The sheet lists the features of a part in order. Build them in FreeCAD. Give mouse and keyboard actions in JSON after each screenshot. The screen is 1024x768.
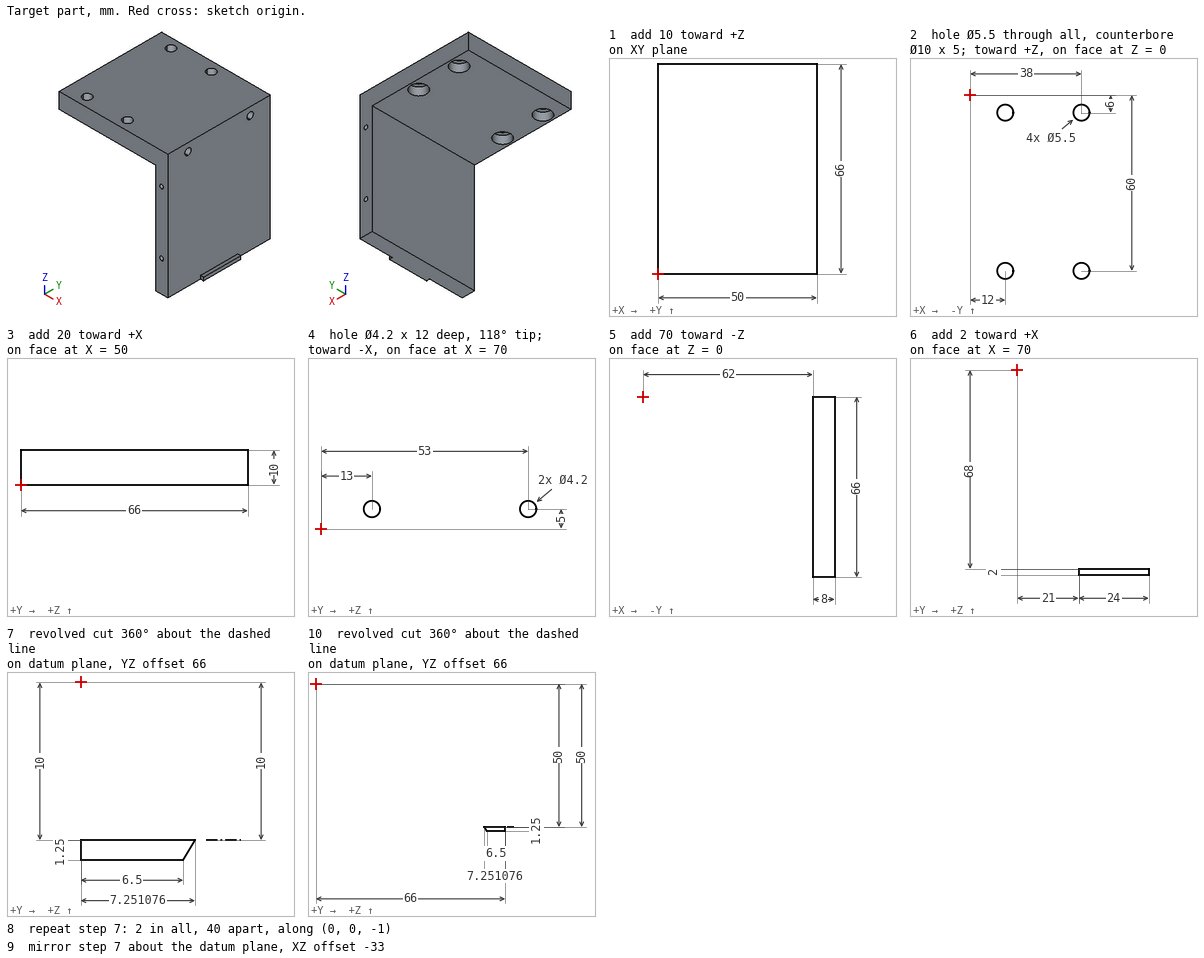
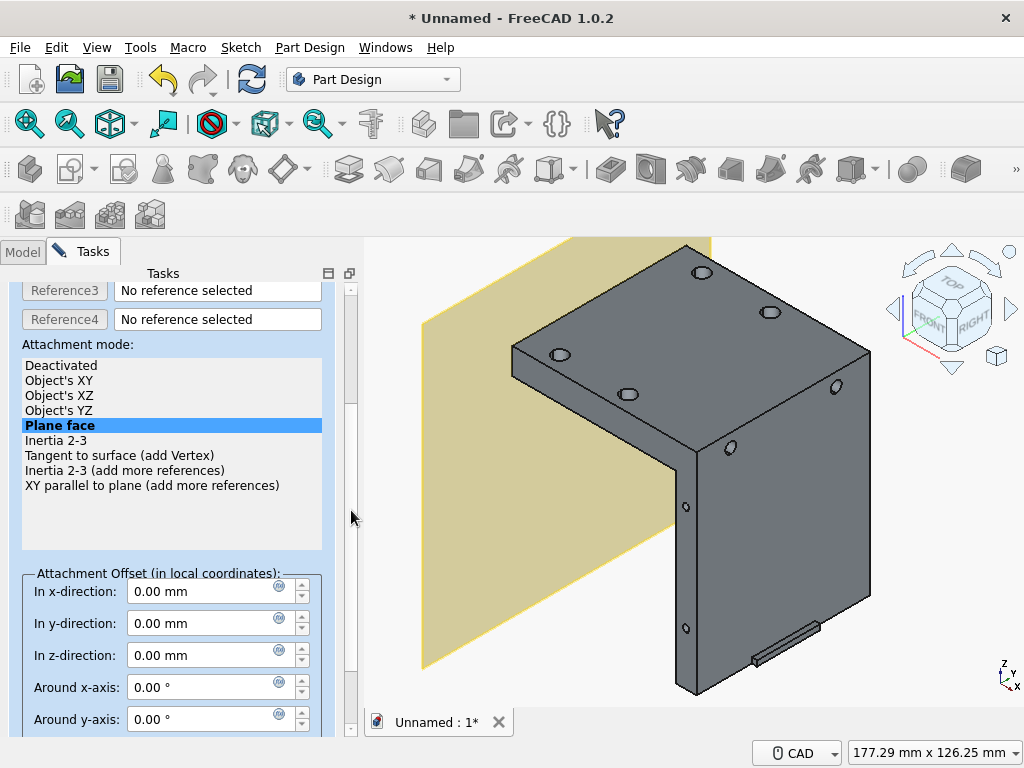
{"action": "triple_click", "coordinate": [210, 655]}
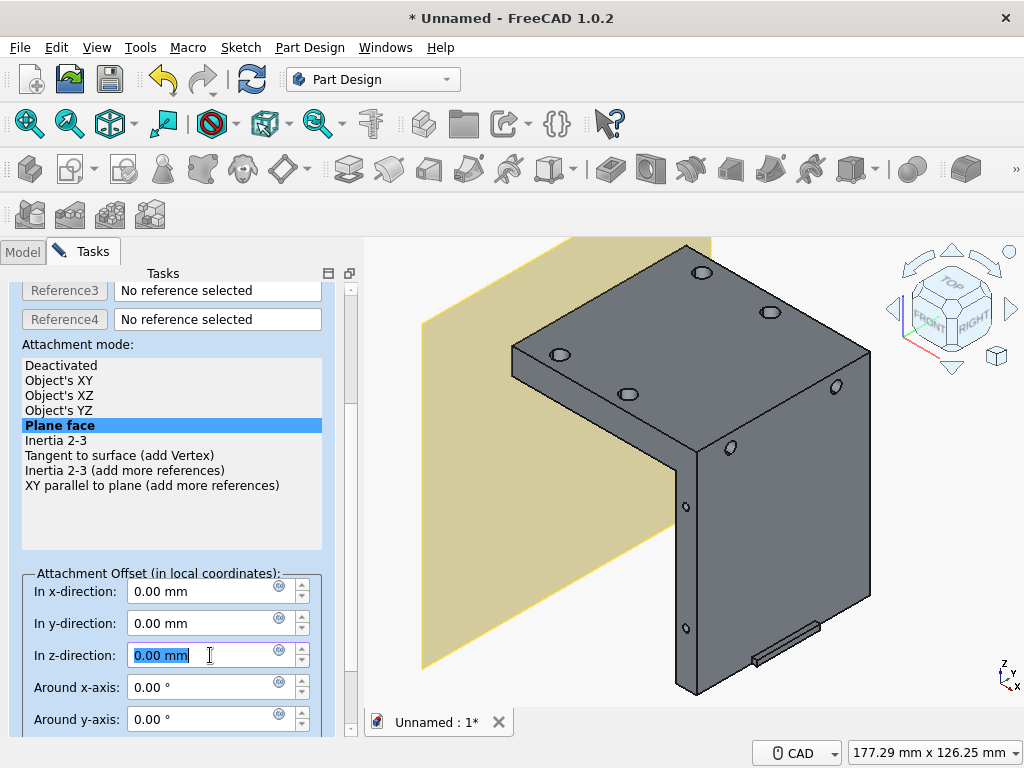
{"action": "type", "text": "66"}
{"action": "key", "text": "Tab"}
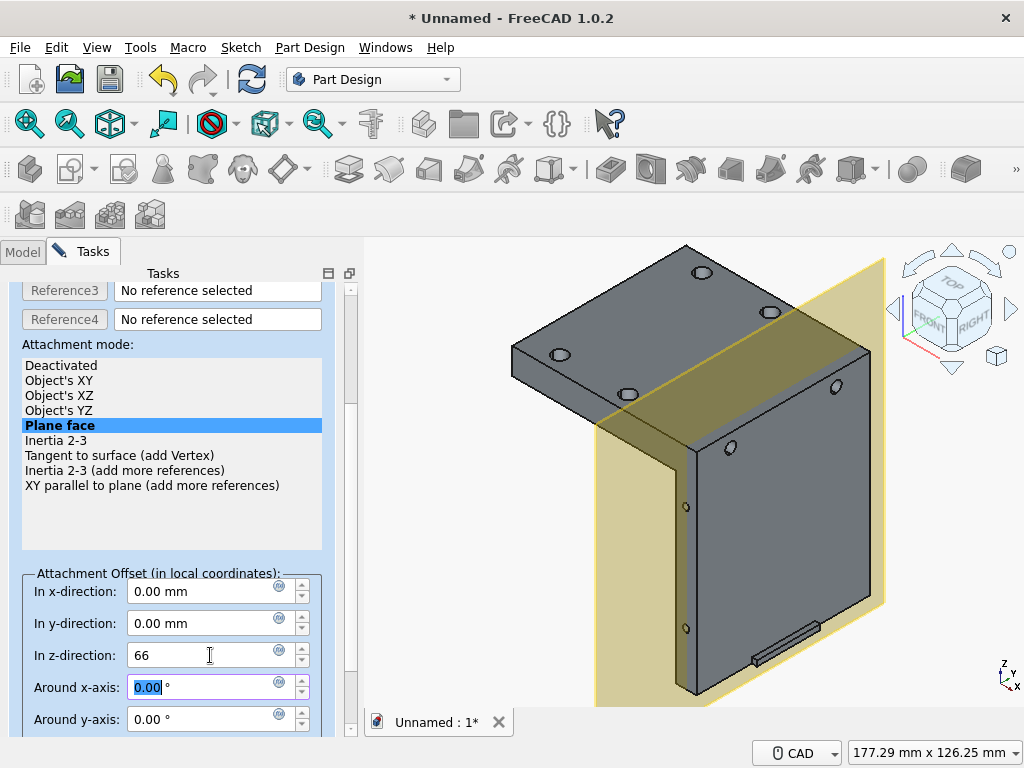
{"action": "scroll", "coordinate": [351, 510], "scroll_direction": "up", "scroll_amount": 4}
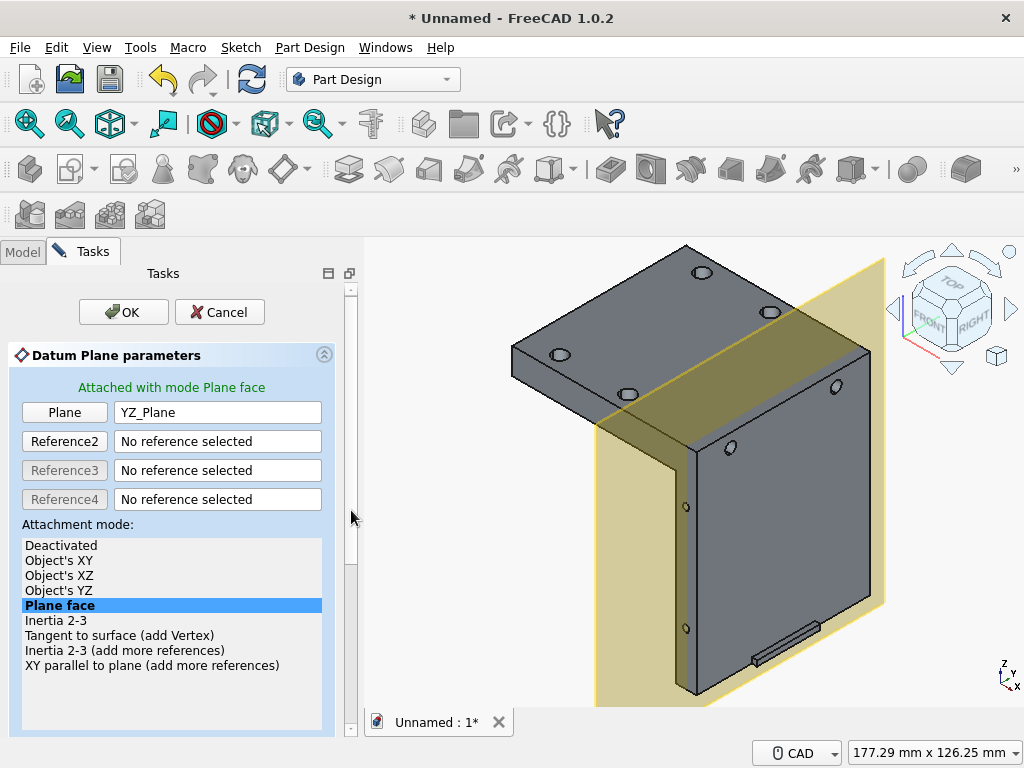
{"action": "left_click", "coordinate": [124, 312]}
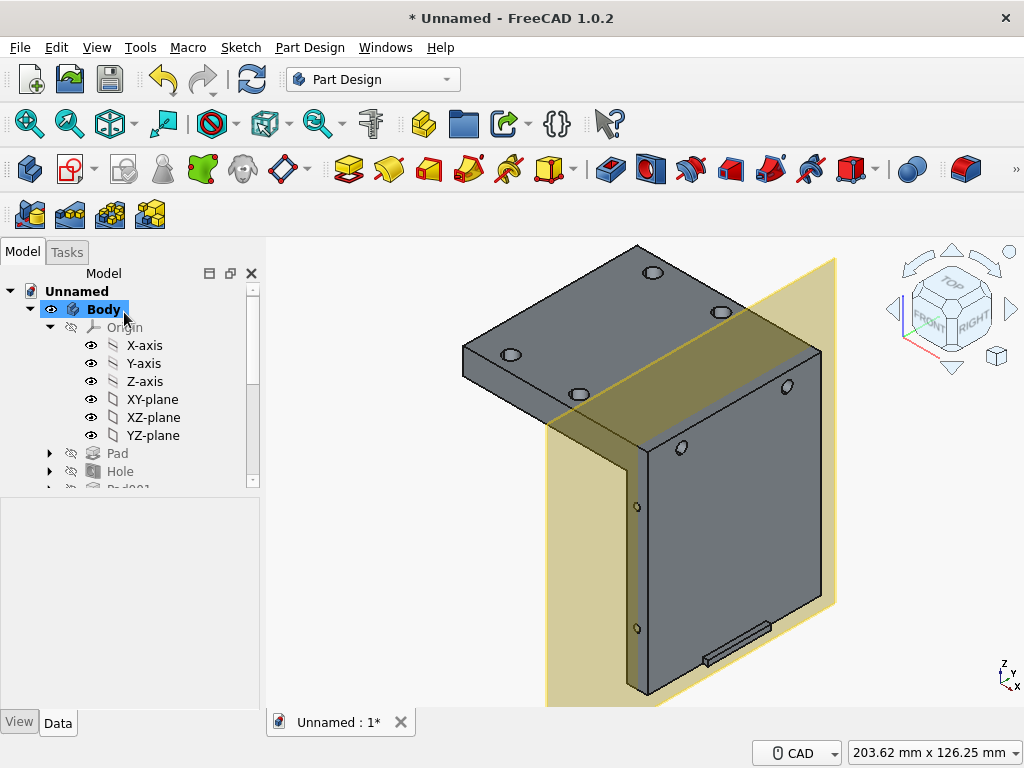
{"action": "scroll", "coordinate": [100, 377], "scroll_direction": "down", "scroll_amount": 3}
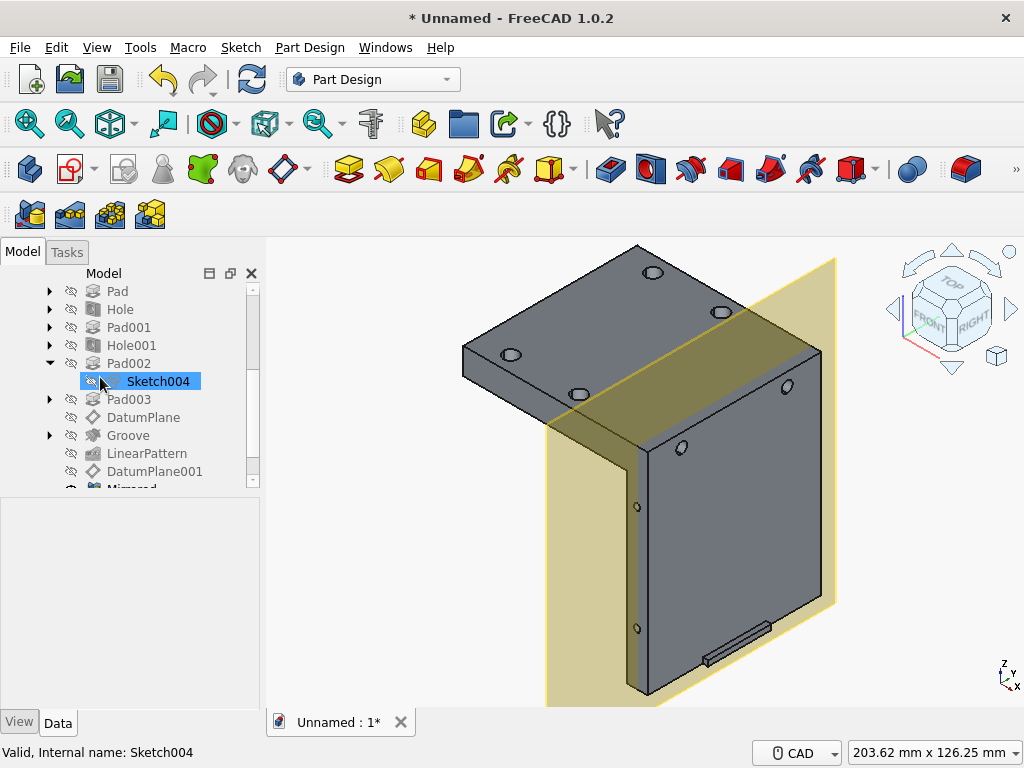
{"action": "scroll", "coordinate": [140, 377], "scroll_direction": "up", "scroll_amount": 15}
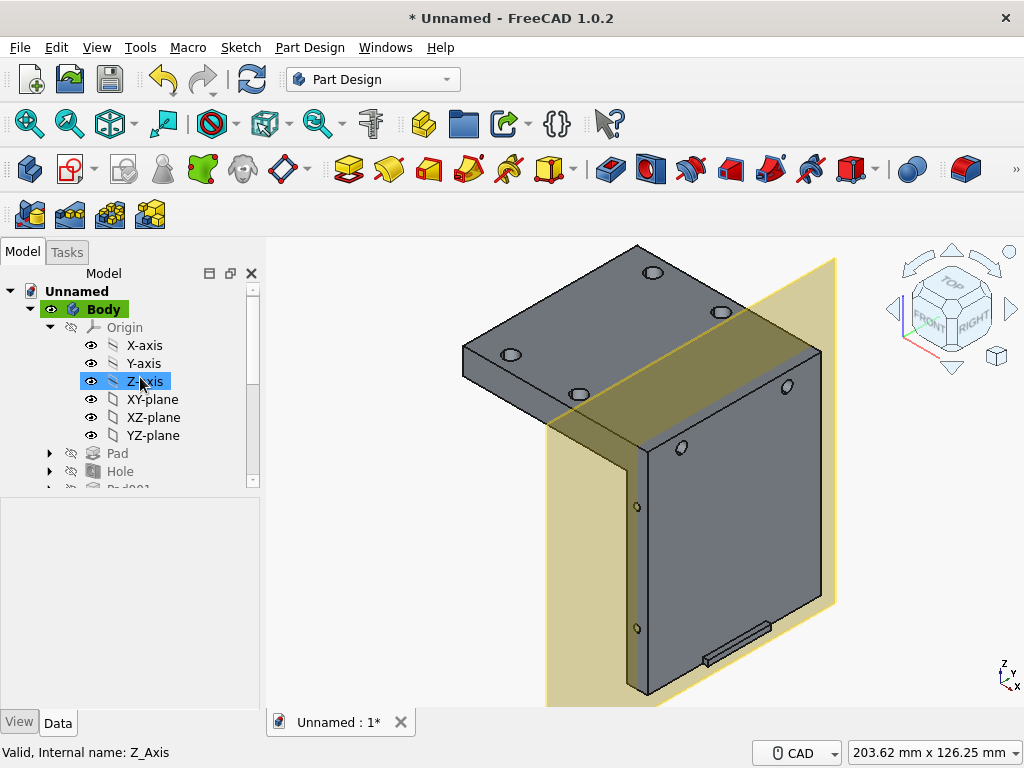
{"action": "scroll", "coordinate": [100, 377], "scroll_direction": "down", "scroll_amount": 6}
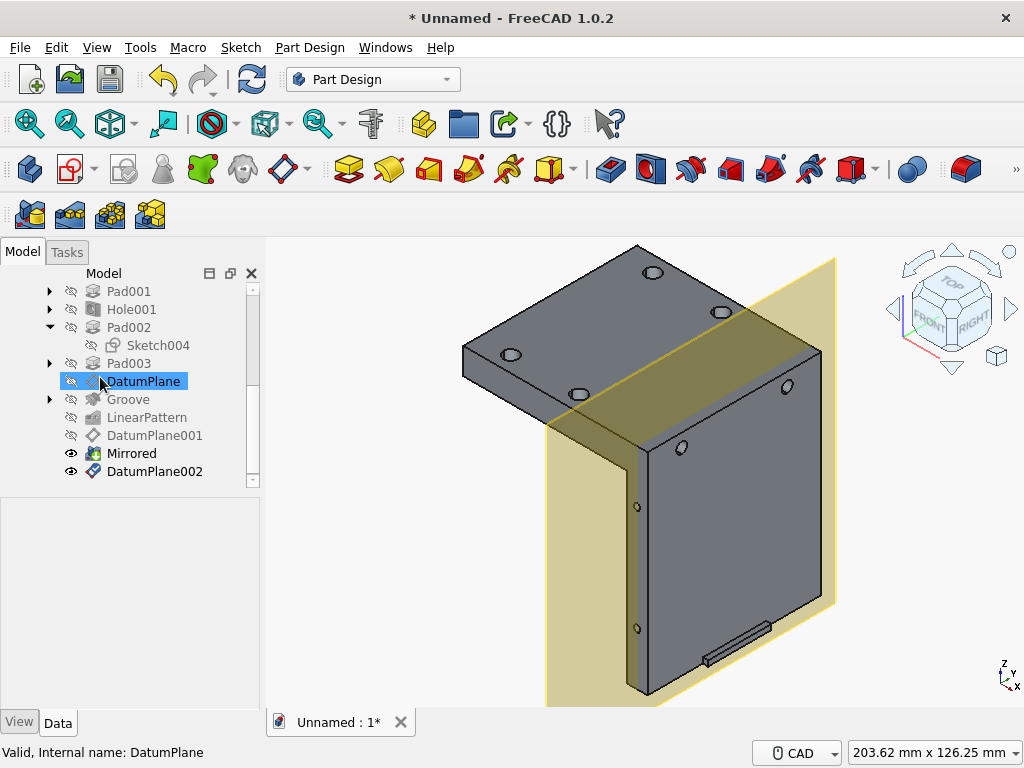
{"action": "left_click", "coordinate": [116, 471]}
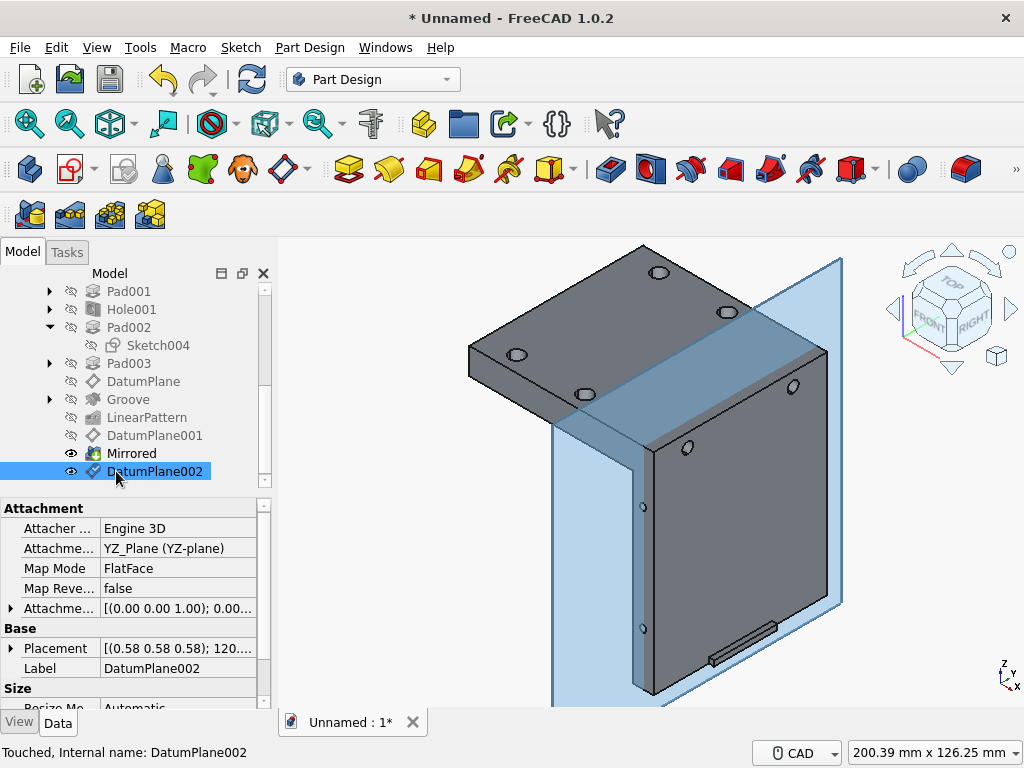
{"action": "left_click", "coordinate": [70, 170]}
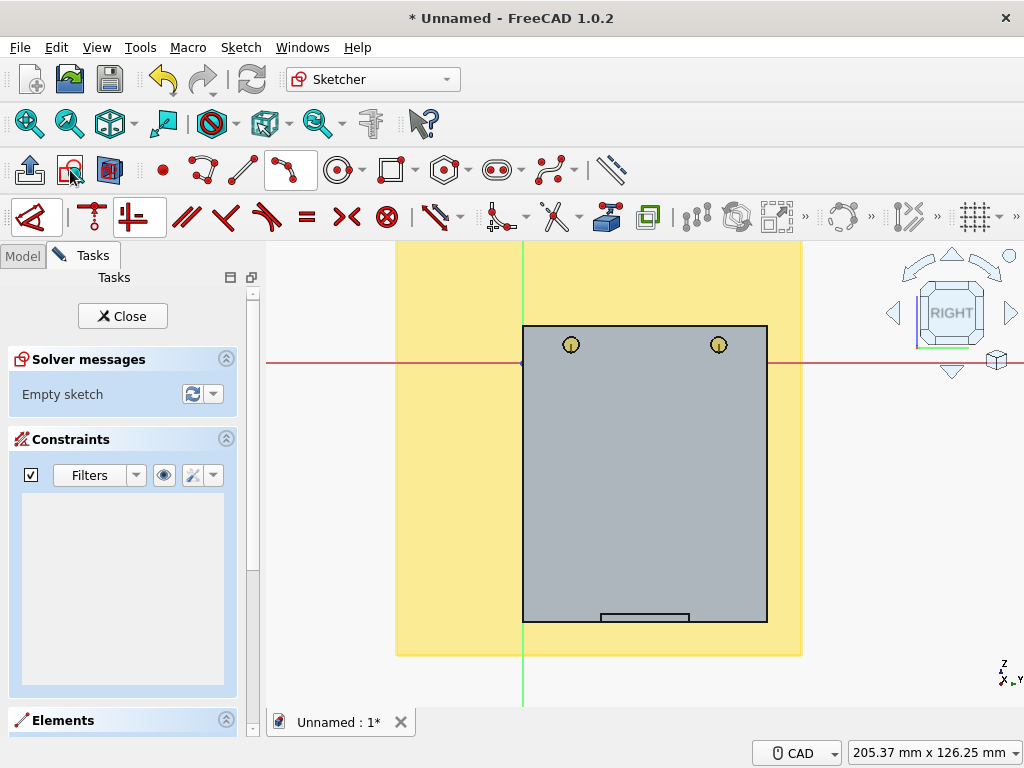
{"action": "key", "text": "q s"}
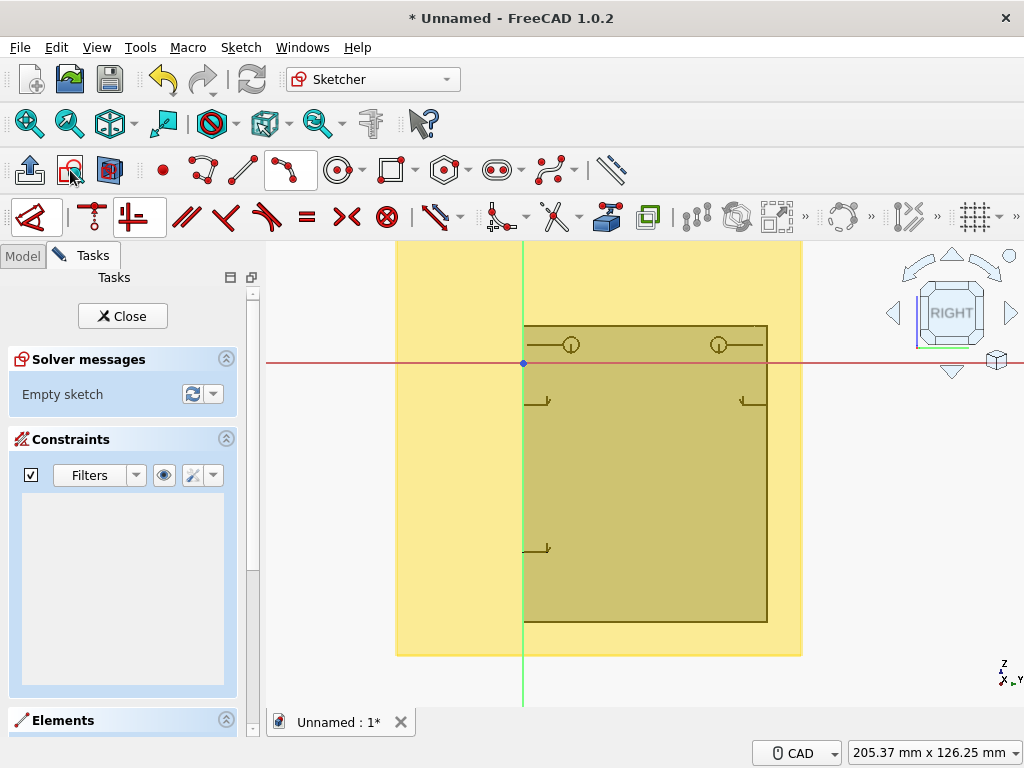
{"action": "scroll", "coordinate": [777, 558], "scroll_direction": "up", "scroll_amount": 12}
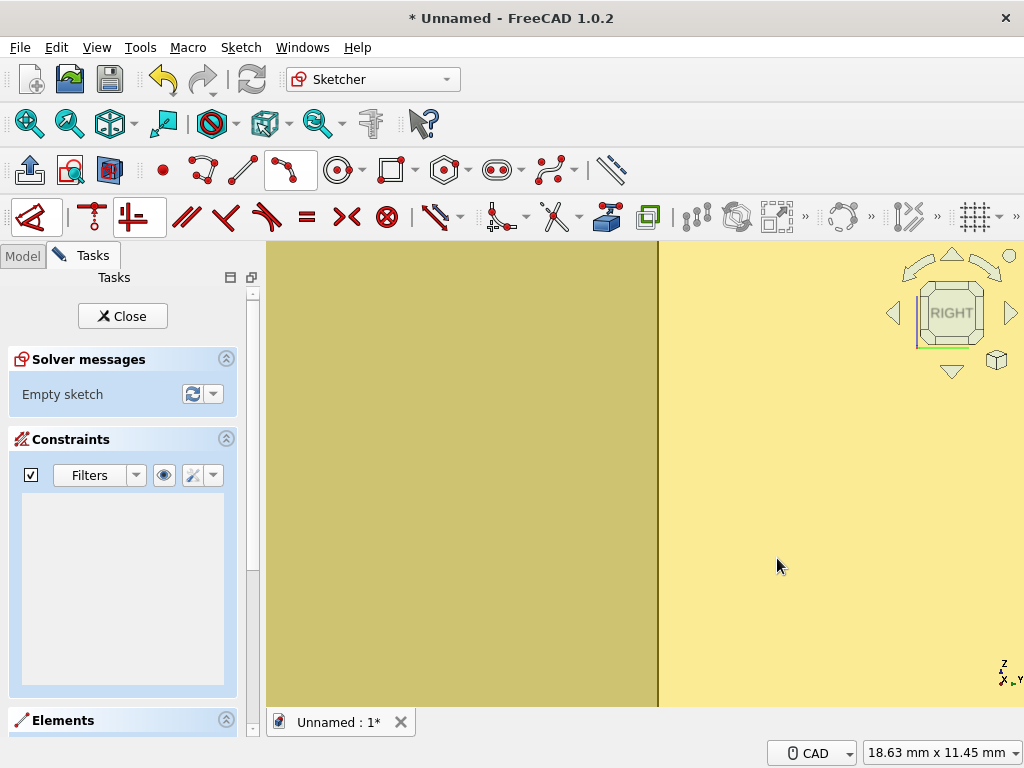
{"action": "left_click", "coordinate": [204, 170]}